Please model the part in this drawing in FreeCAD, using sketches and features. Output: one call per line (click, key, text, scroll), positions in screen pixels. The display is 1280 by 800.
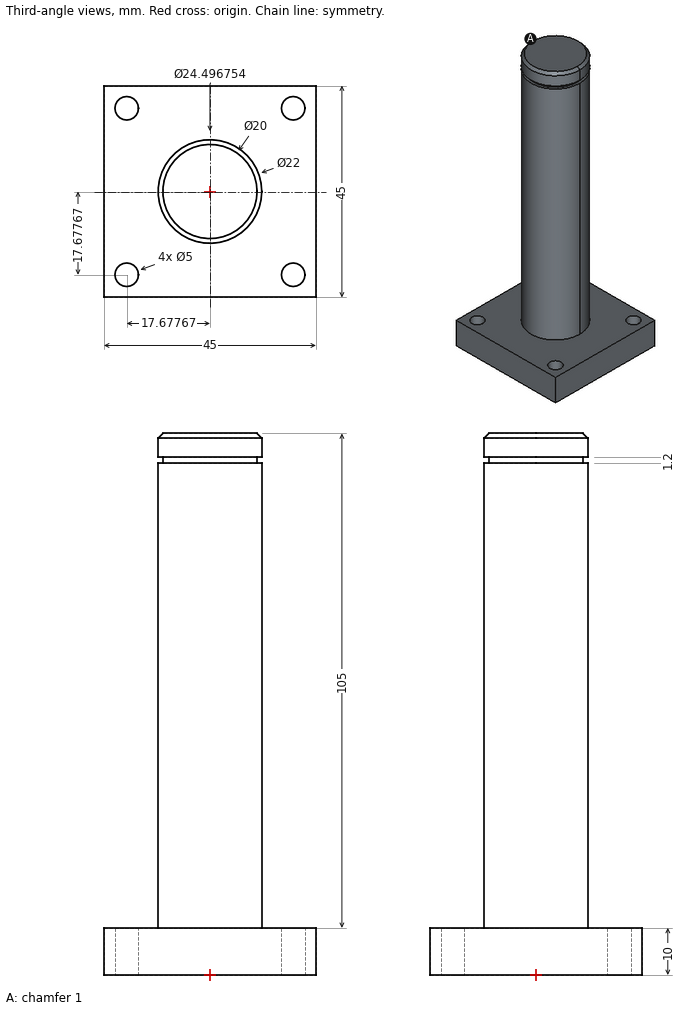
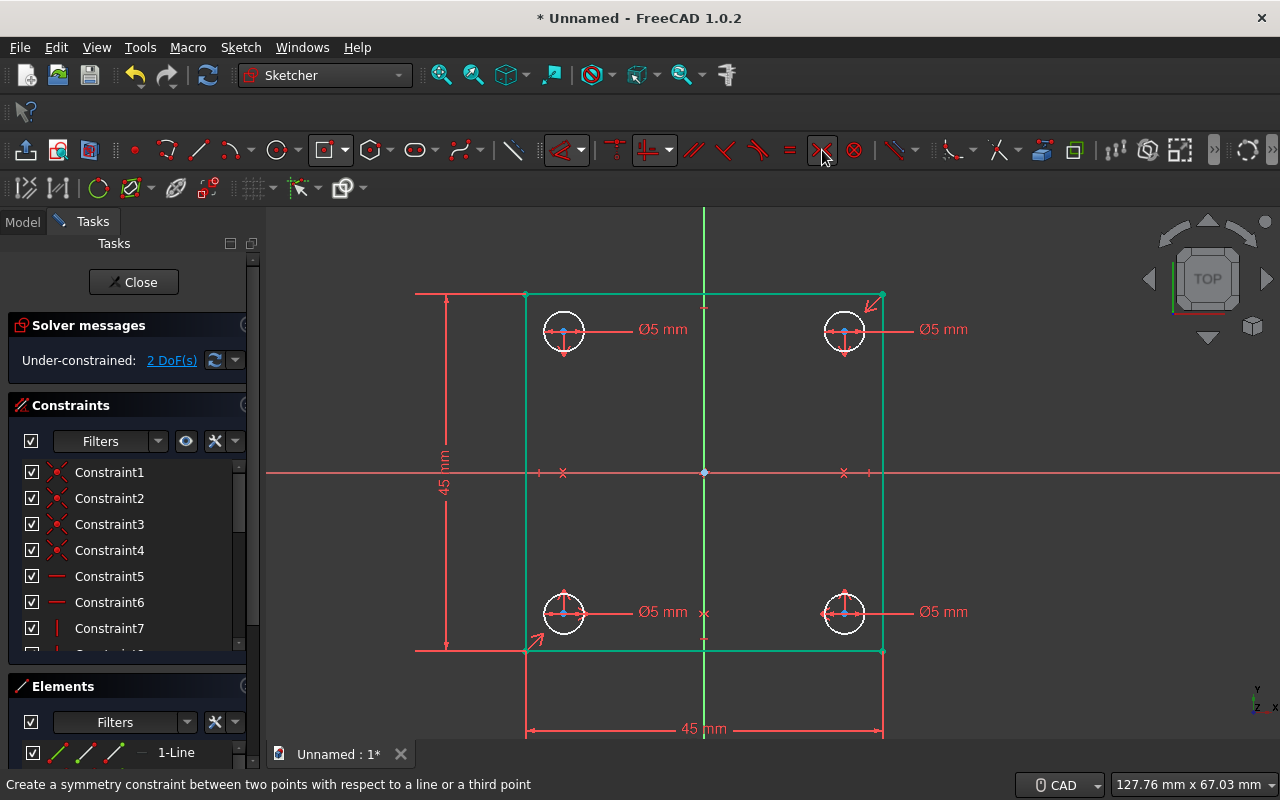
click(564, 614)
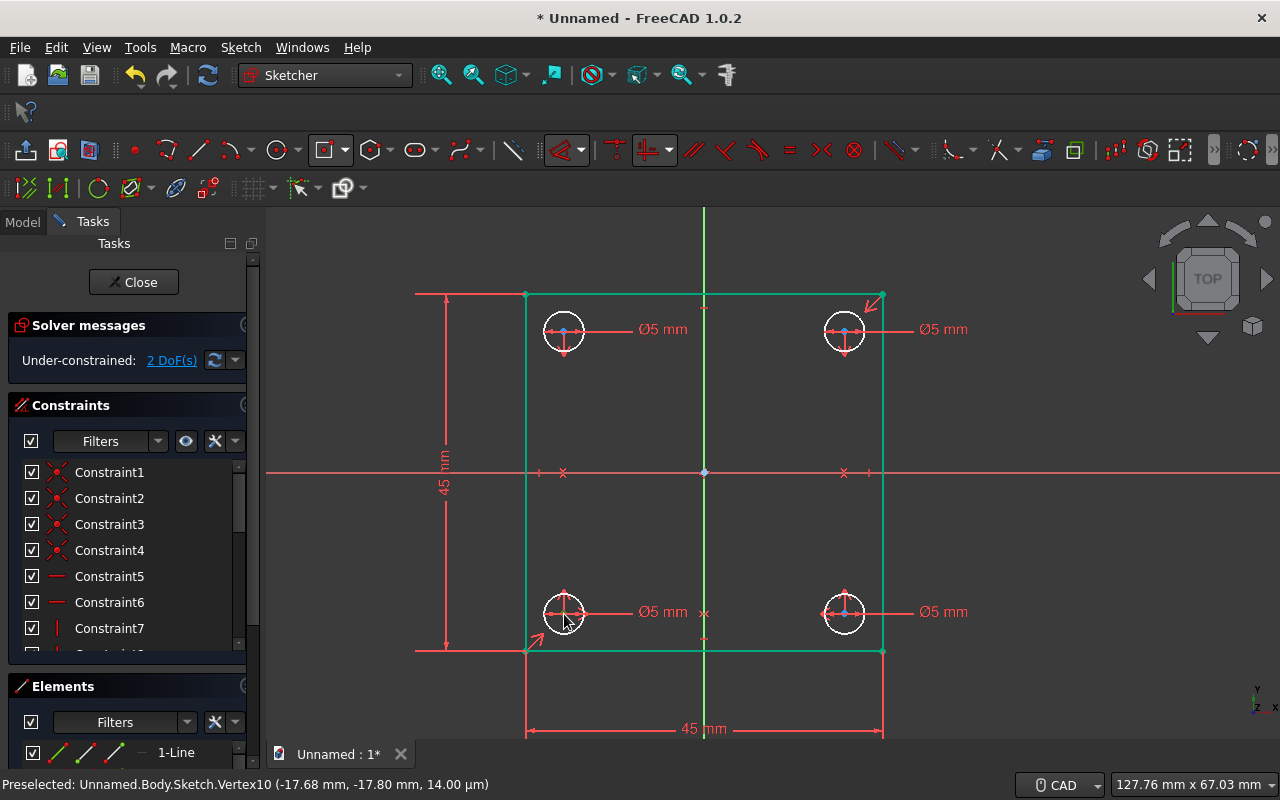
click(584, 150)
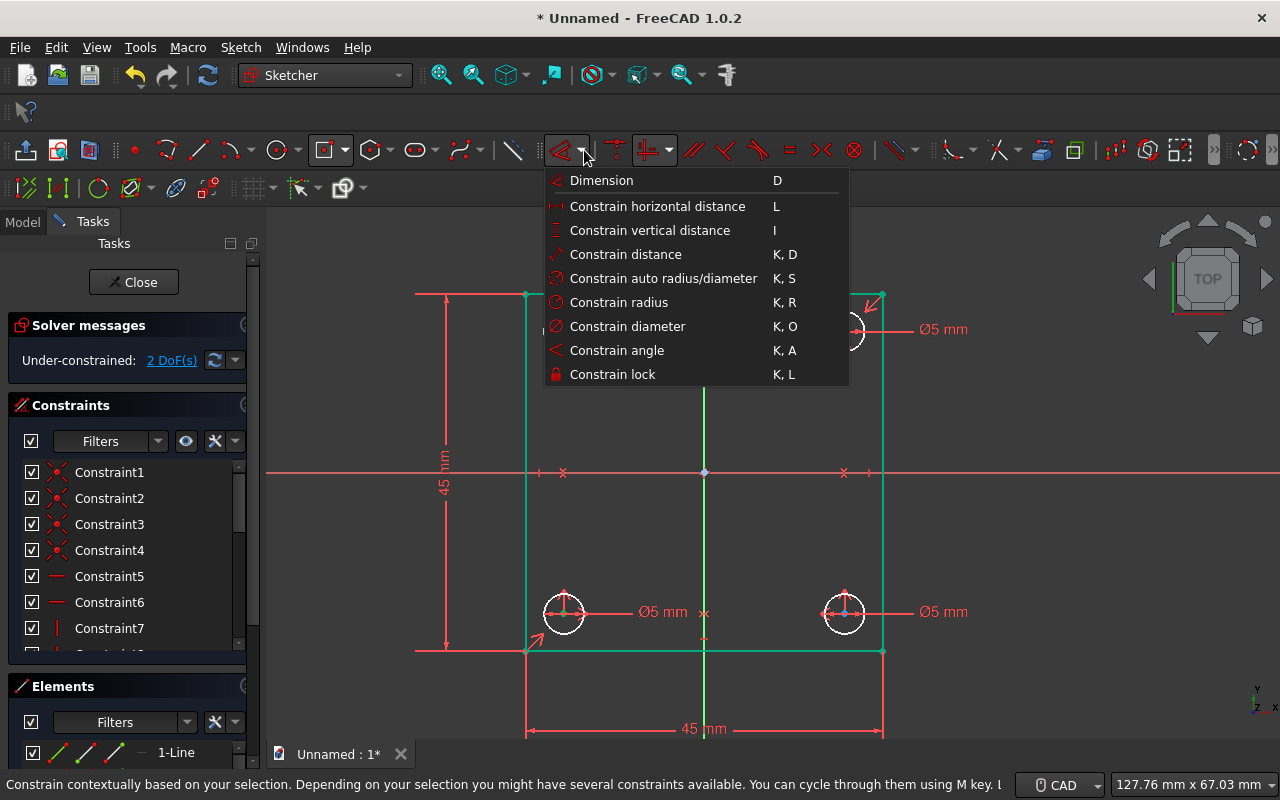
click(697, 206)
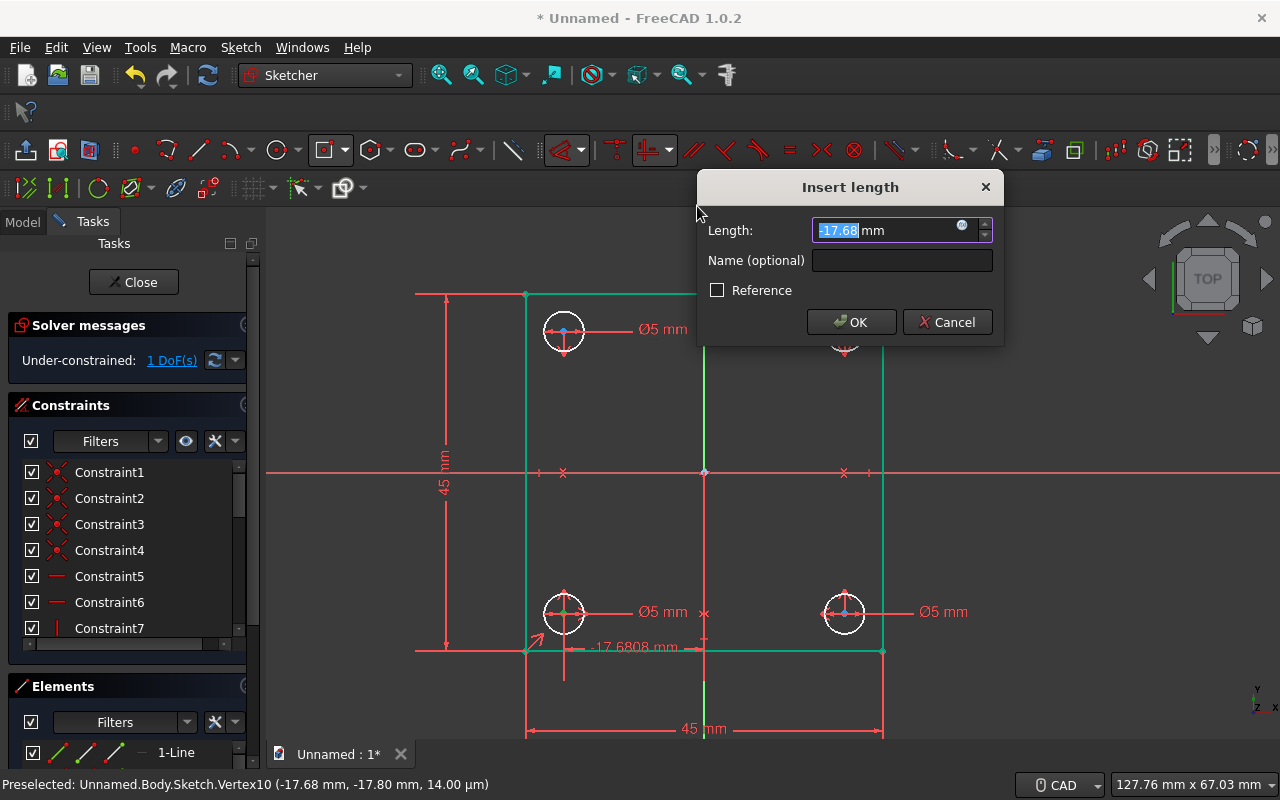
text(-17.67767)
key(Return)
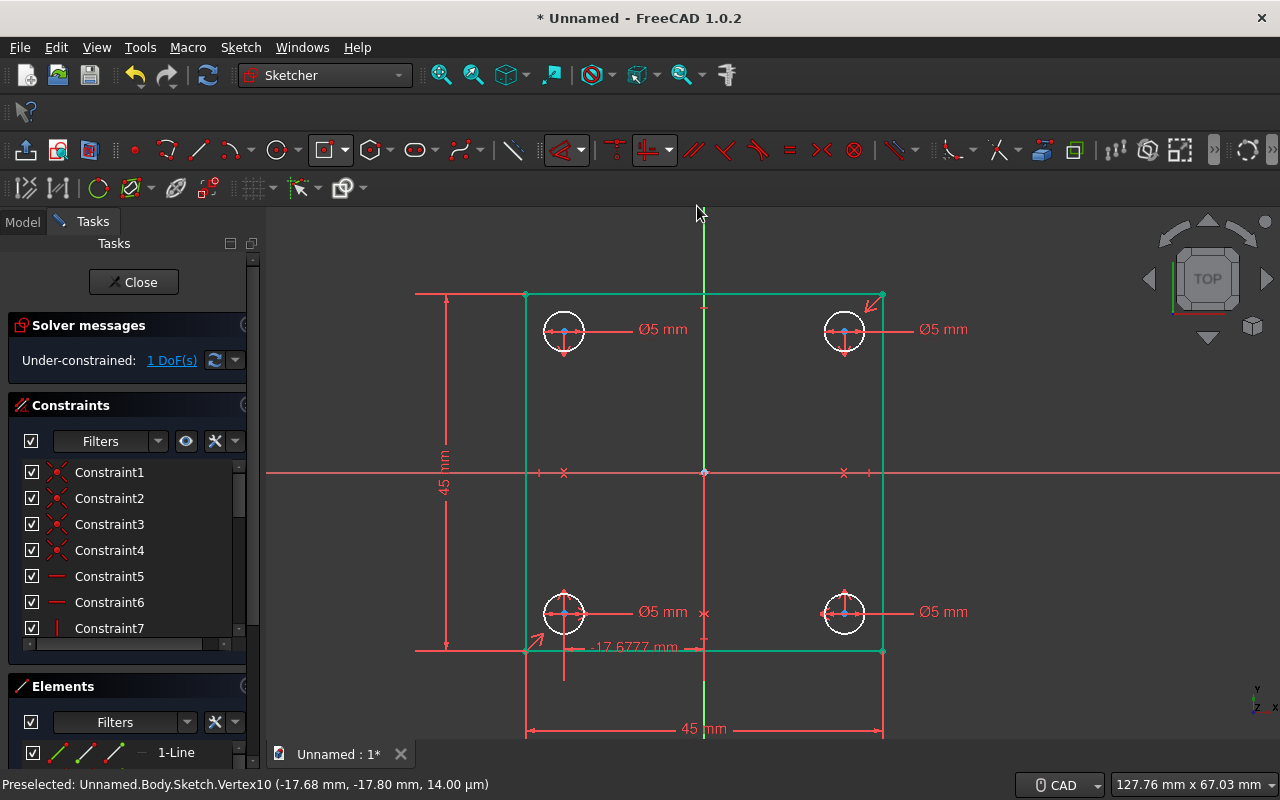
click(564, 614)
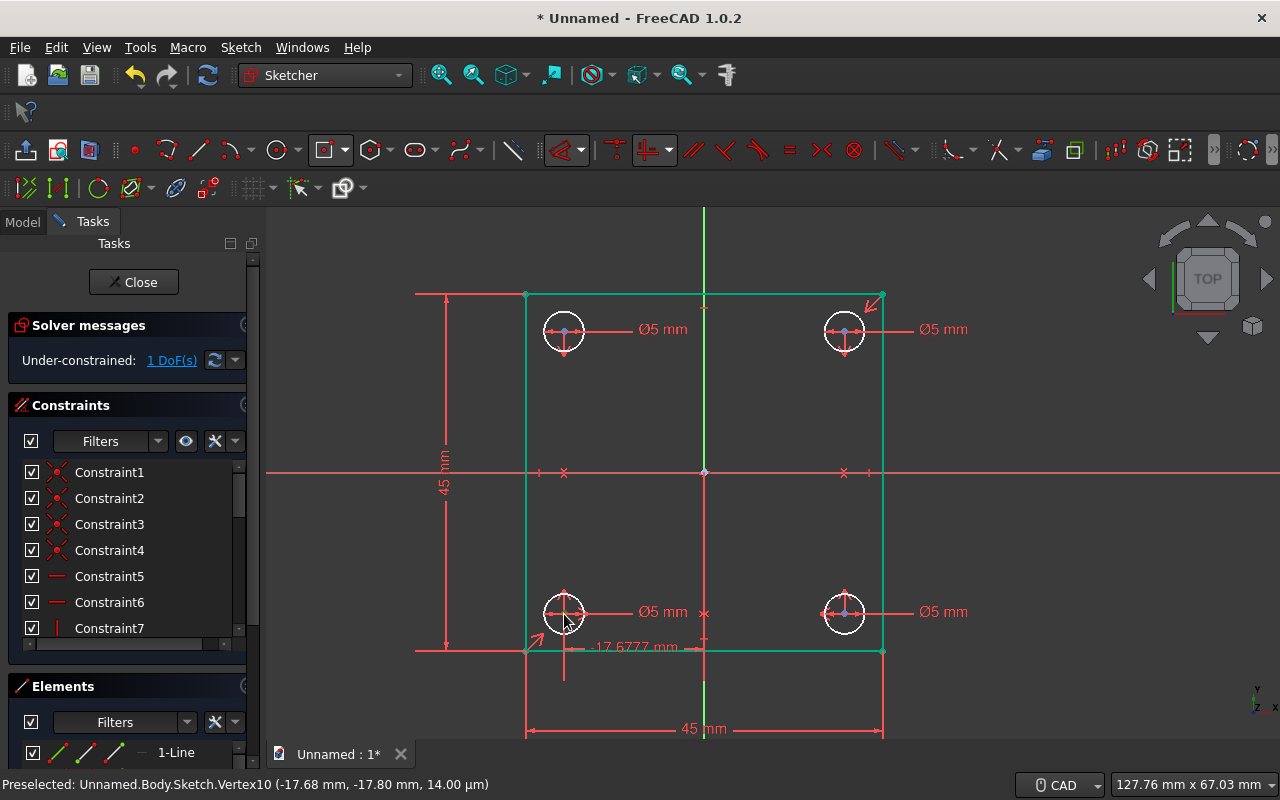
click(584, 150)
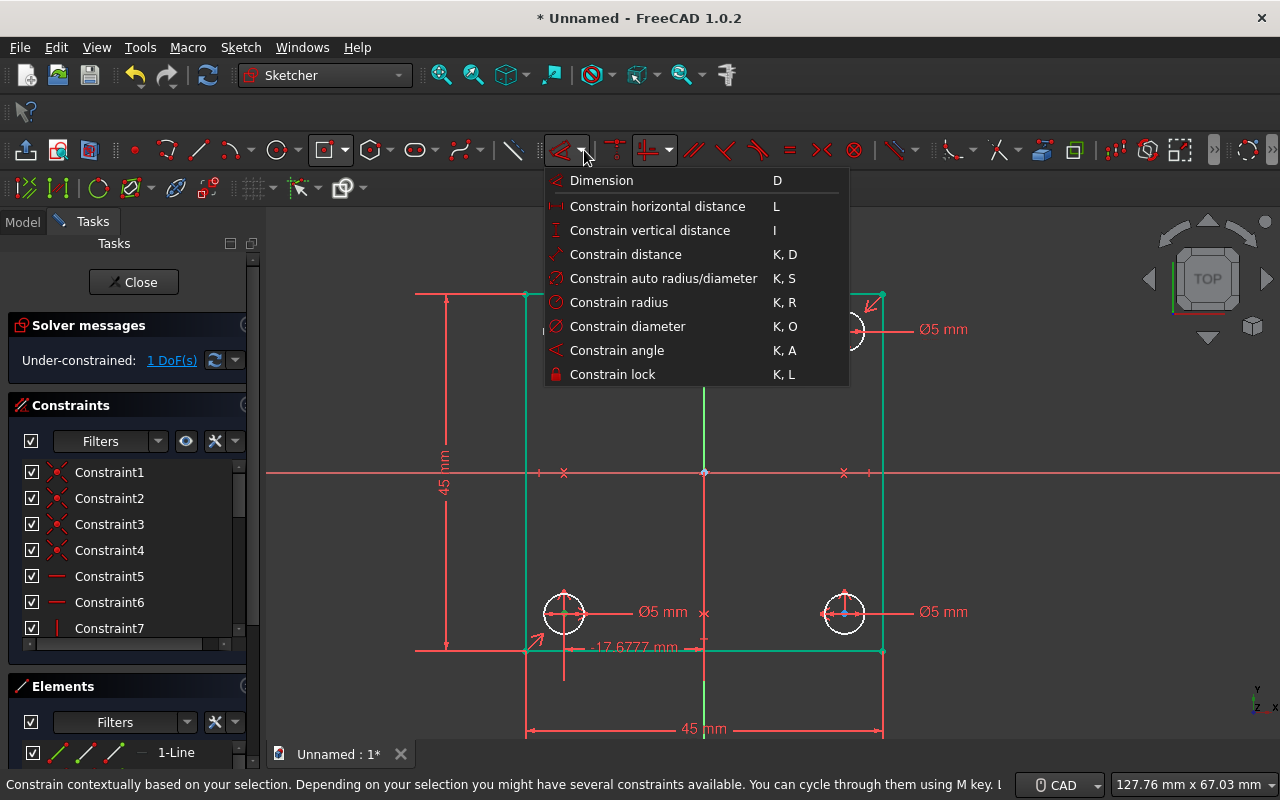
click(697, 230)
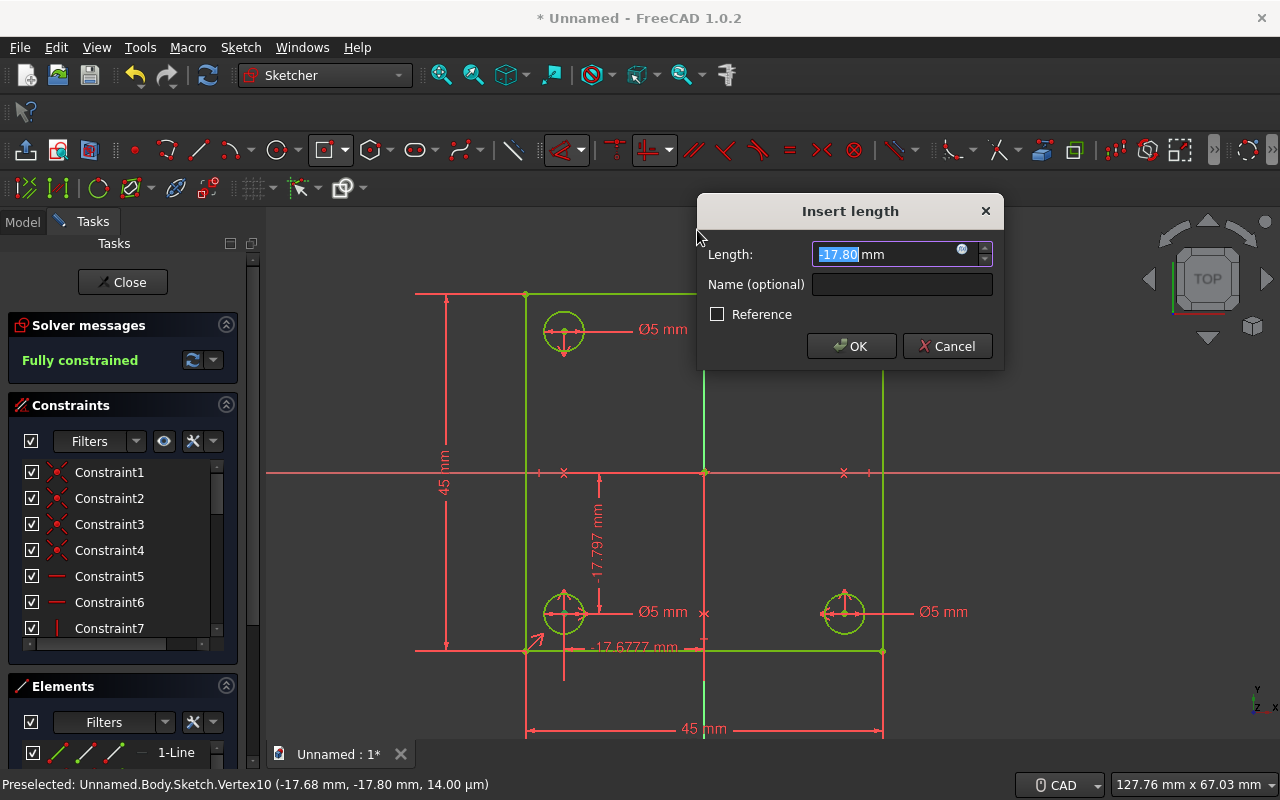
text(-17.67767)
key(Return)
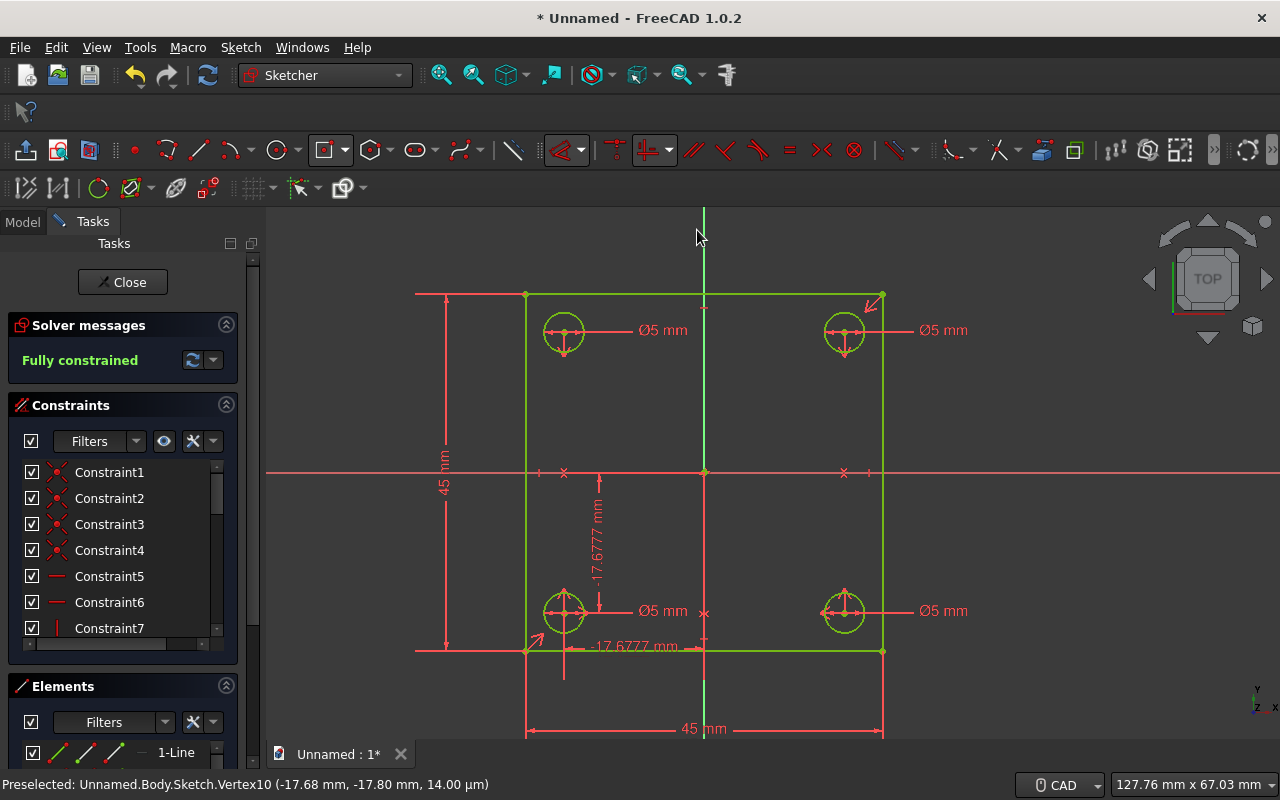
click(123, 282)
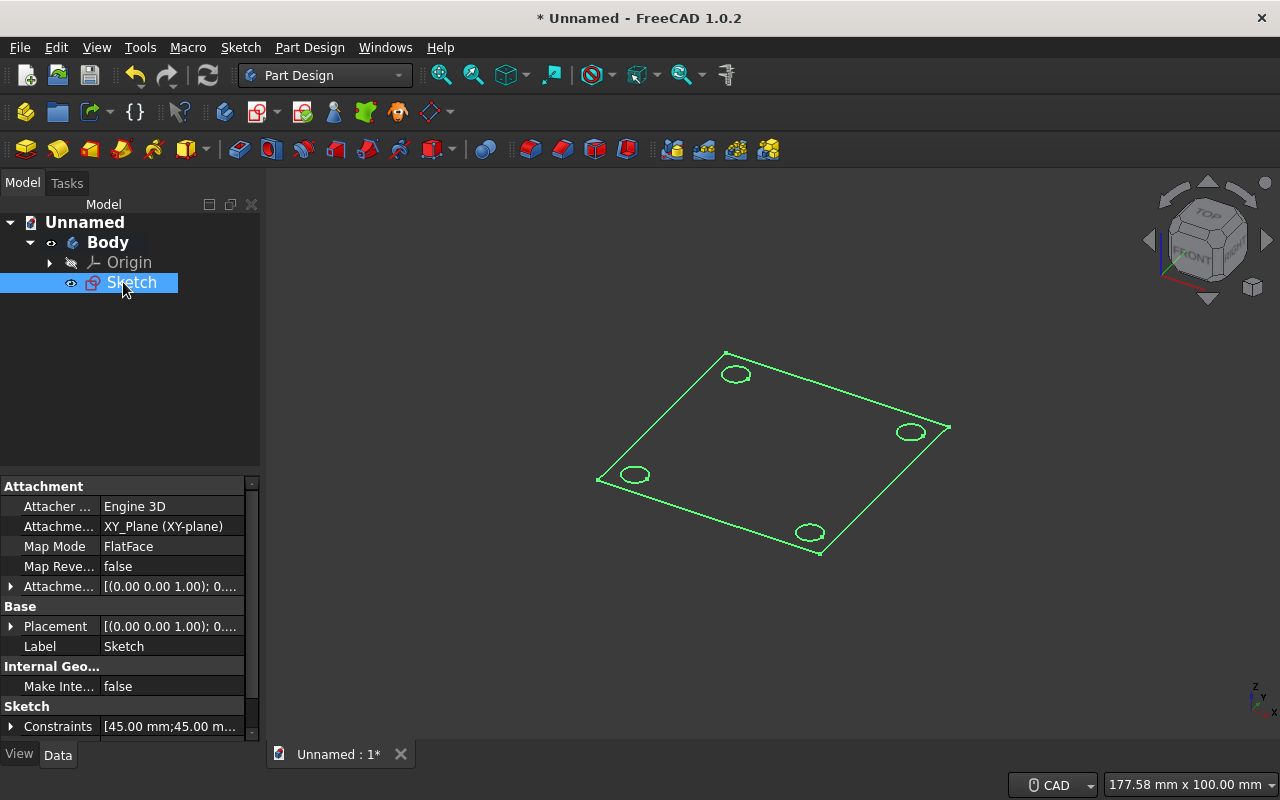
click(26, 150)